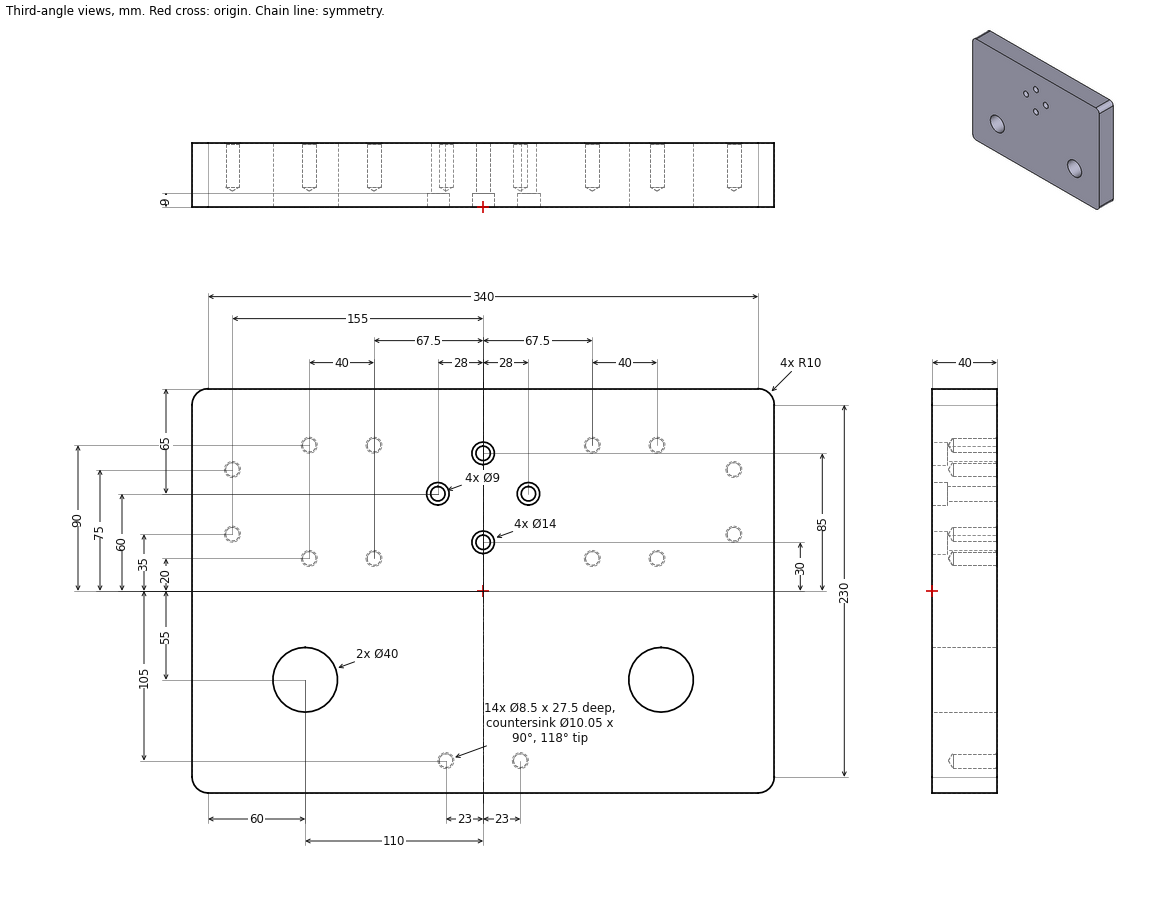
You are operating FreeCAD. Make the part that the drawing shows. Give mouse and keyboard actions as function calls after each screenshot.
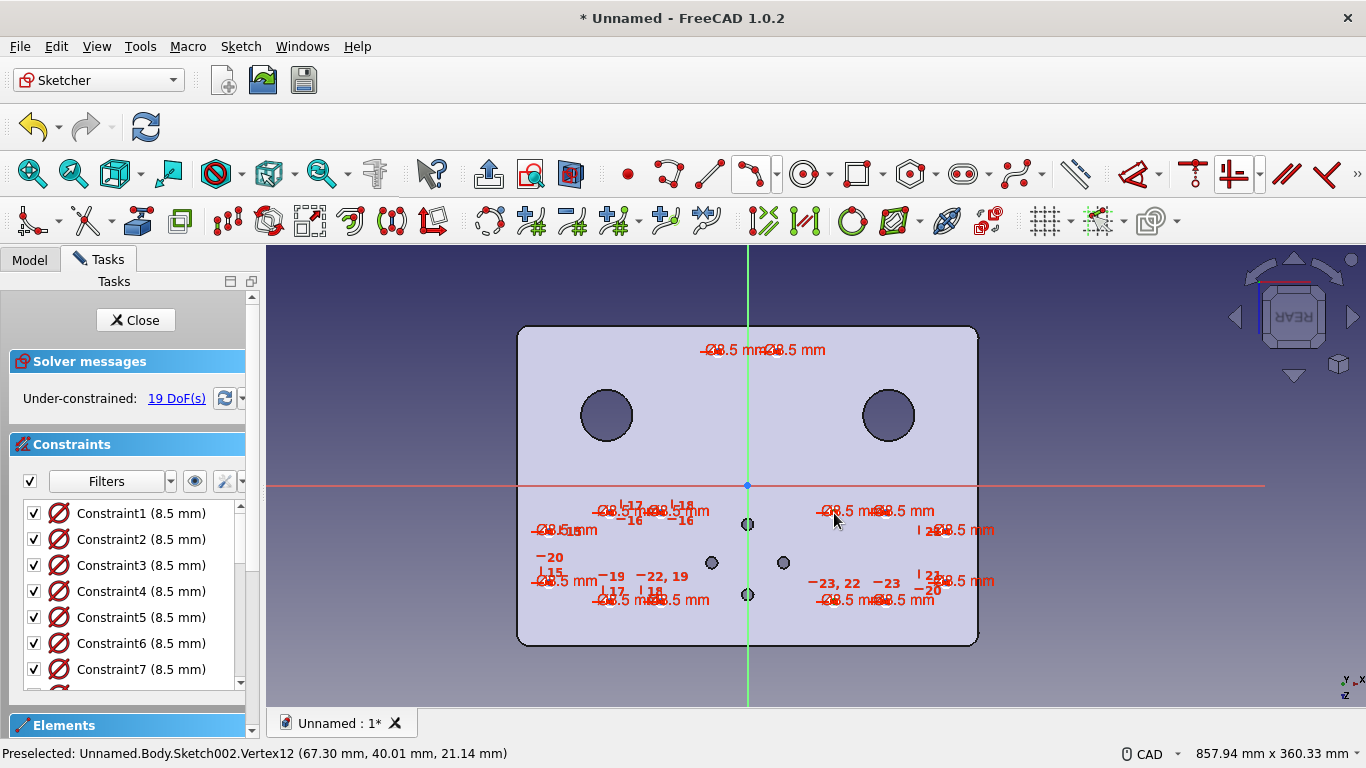
click(1260, 174)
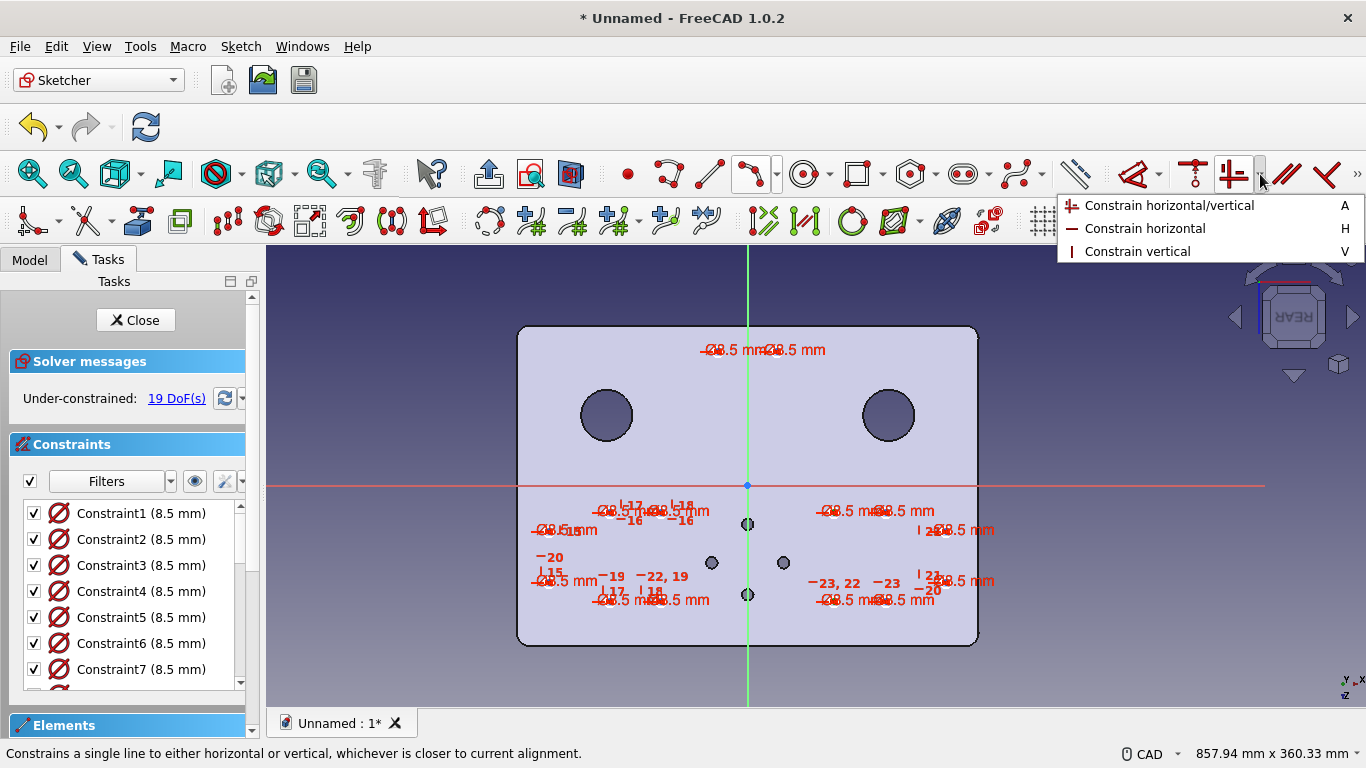
click(1211, 252)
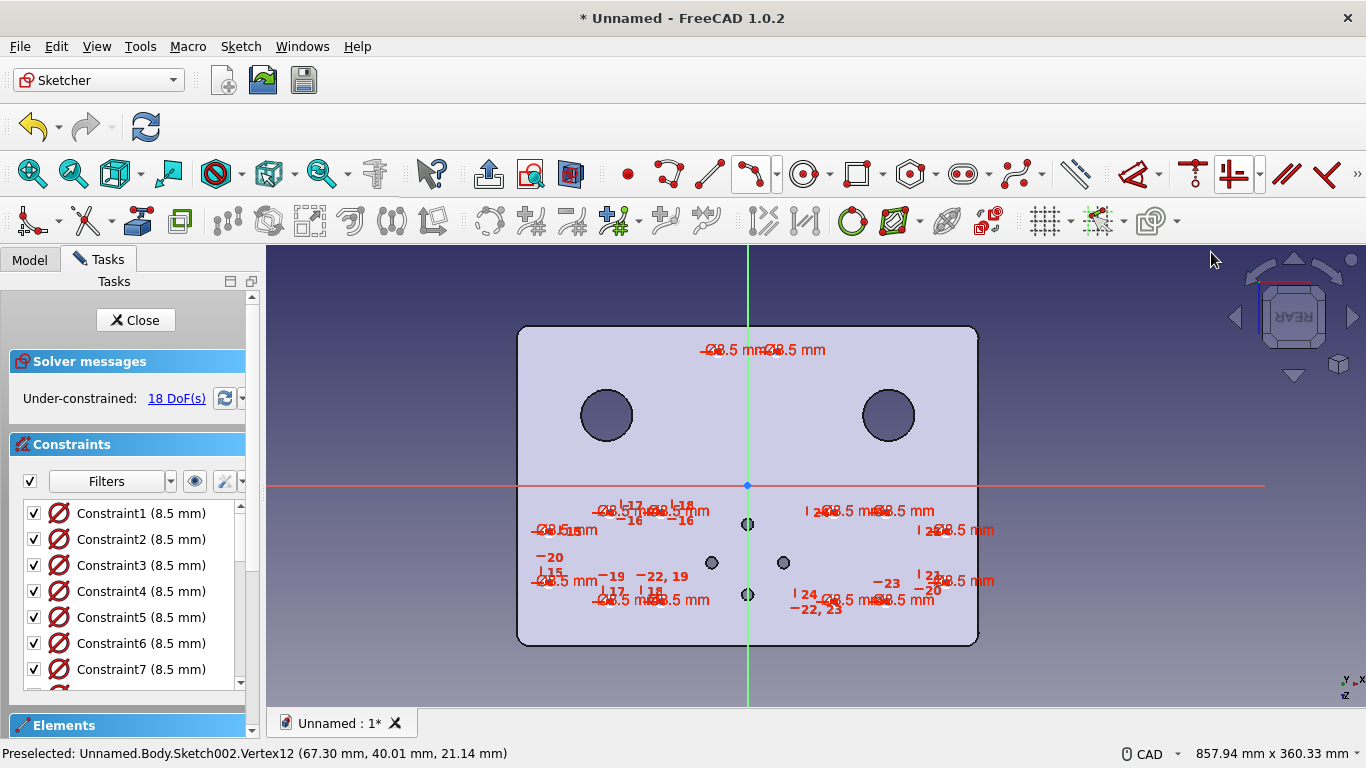
click(661, 513)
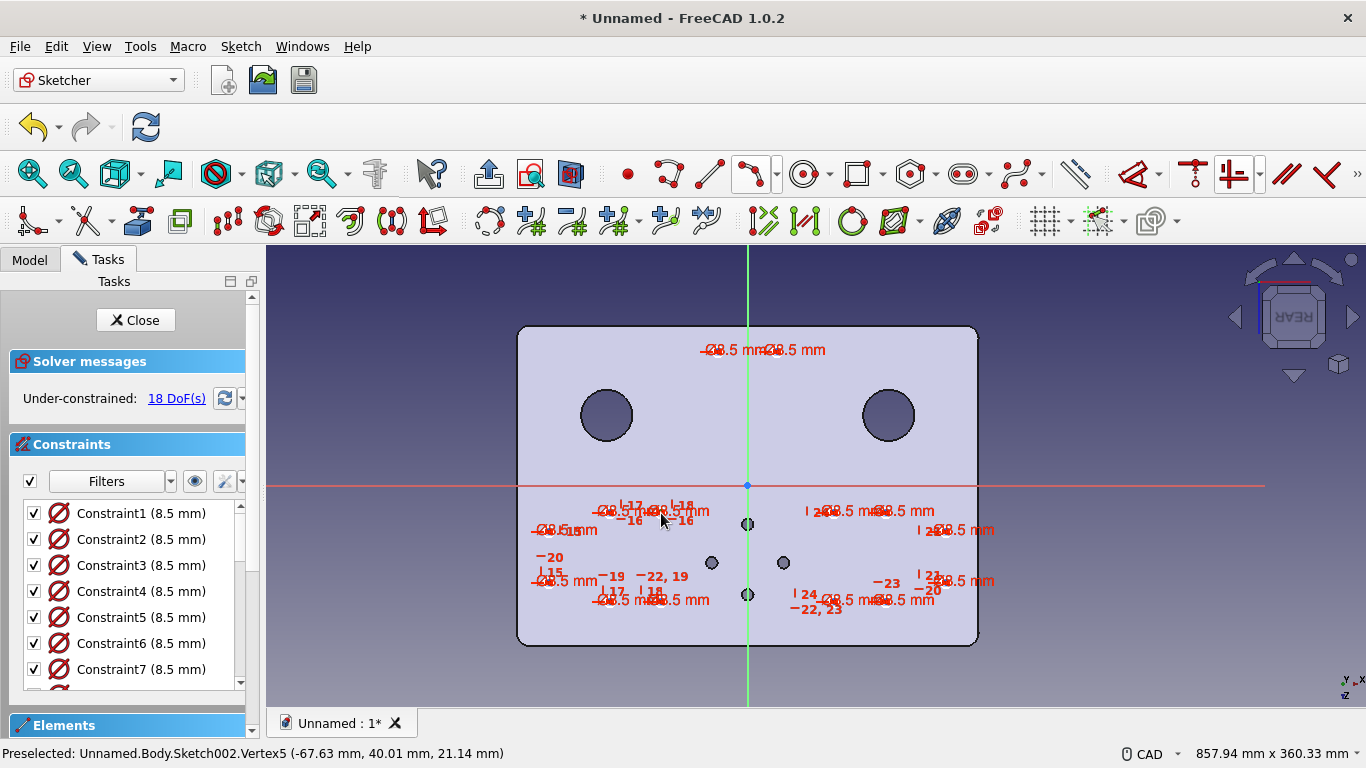
click(834, 513)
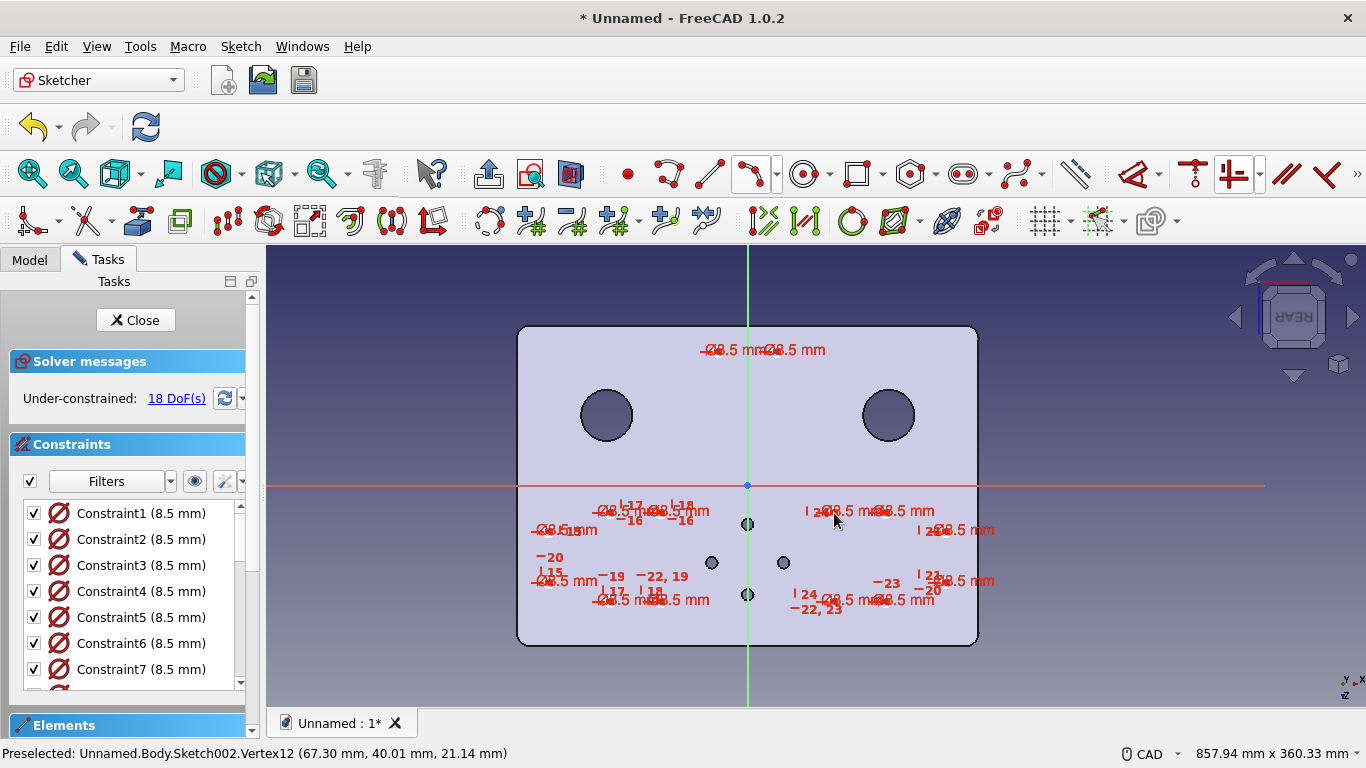
click(1260, 174)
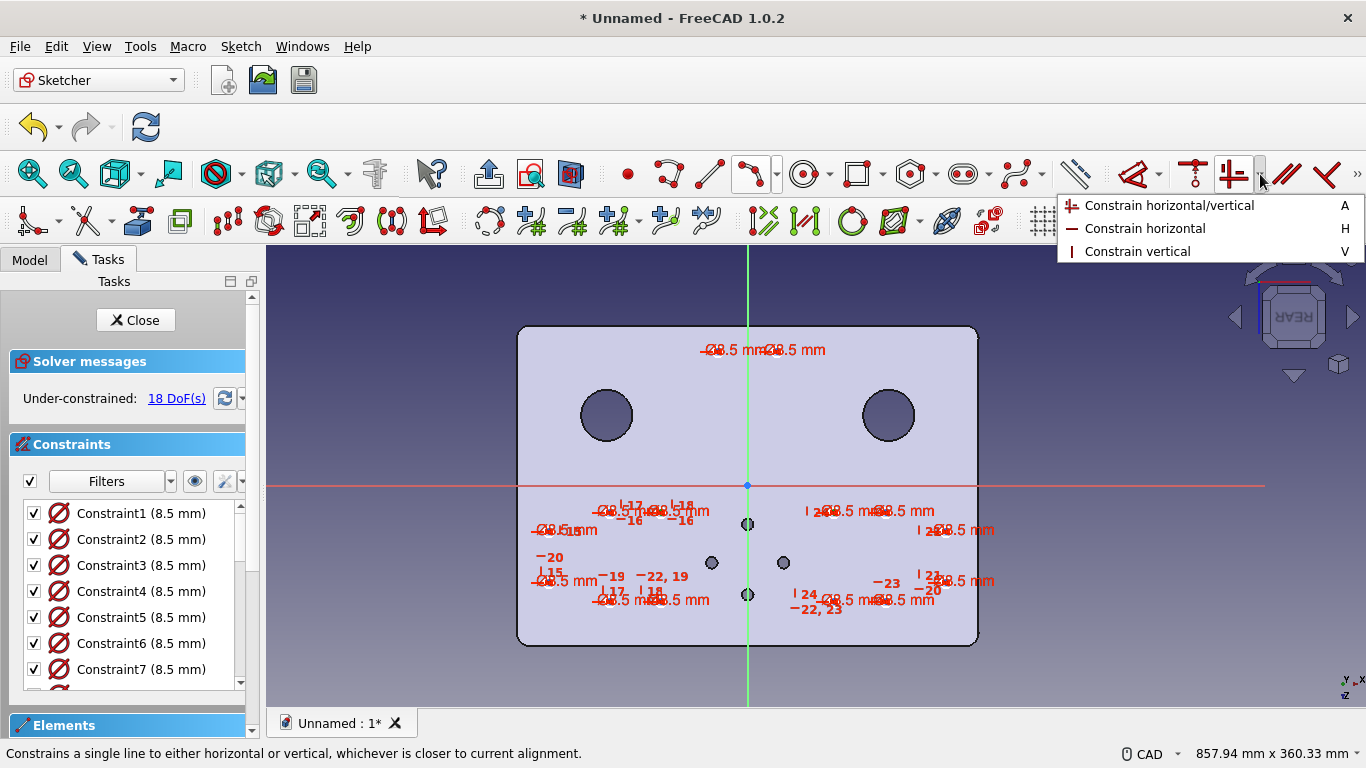
click(1211, 228)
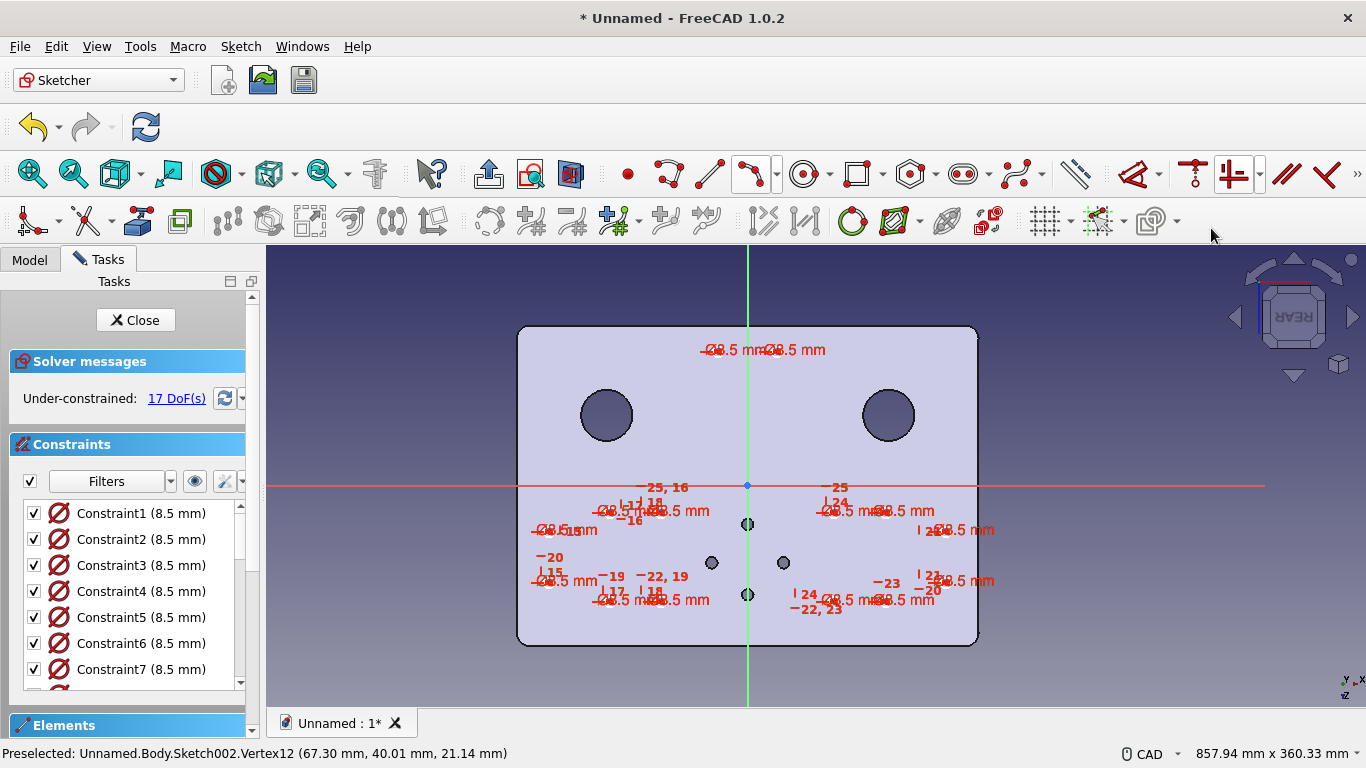
click(886, 602)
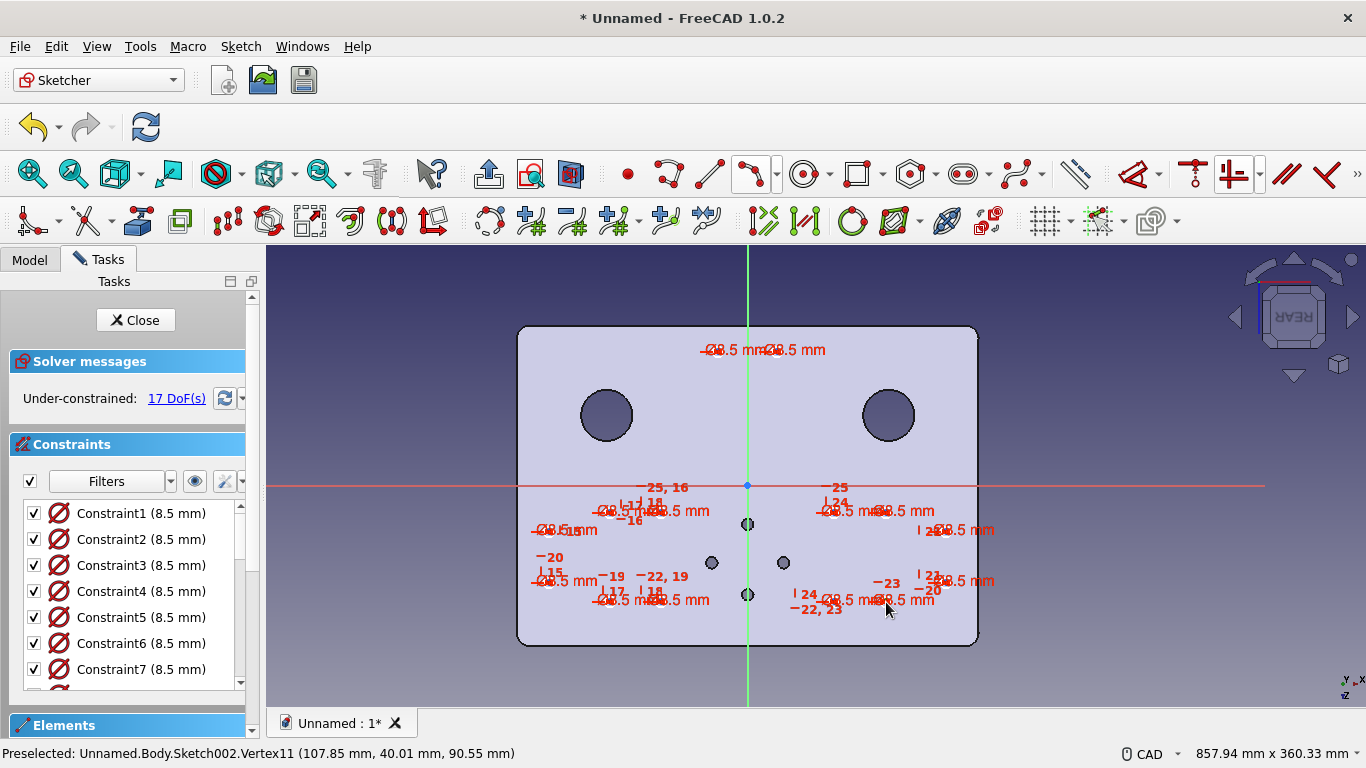
click(886, 513)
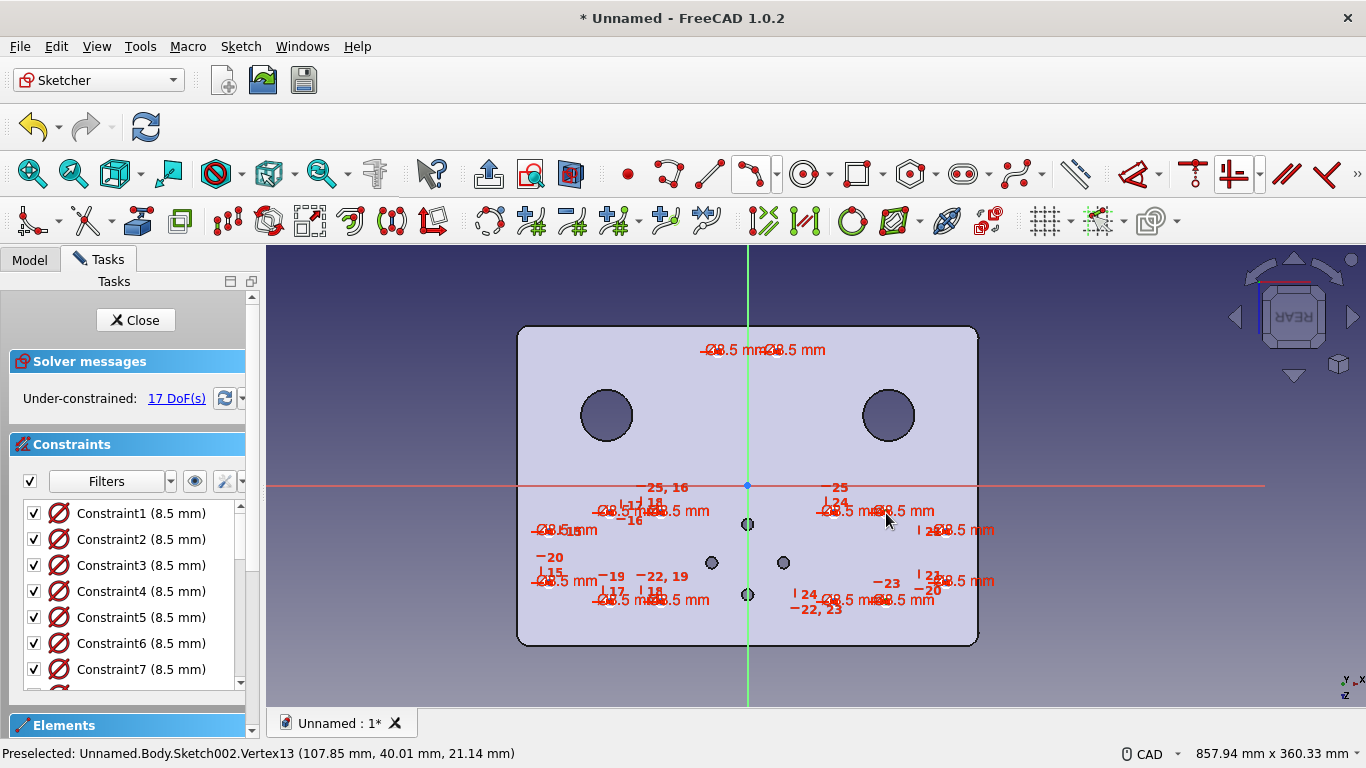
click(1260, 174)